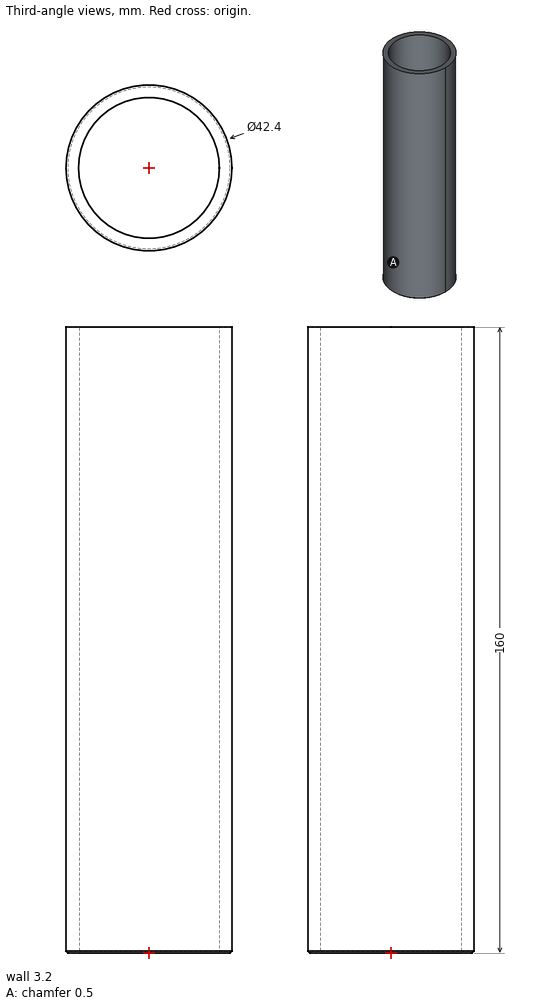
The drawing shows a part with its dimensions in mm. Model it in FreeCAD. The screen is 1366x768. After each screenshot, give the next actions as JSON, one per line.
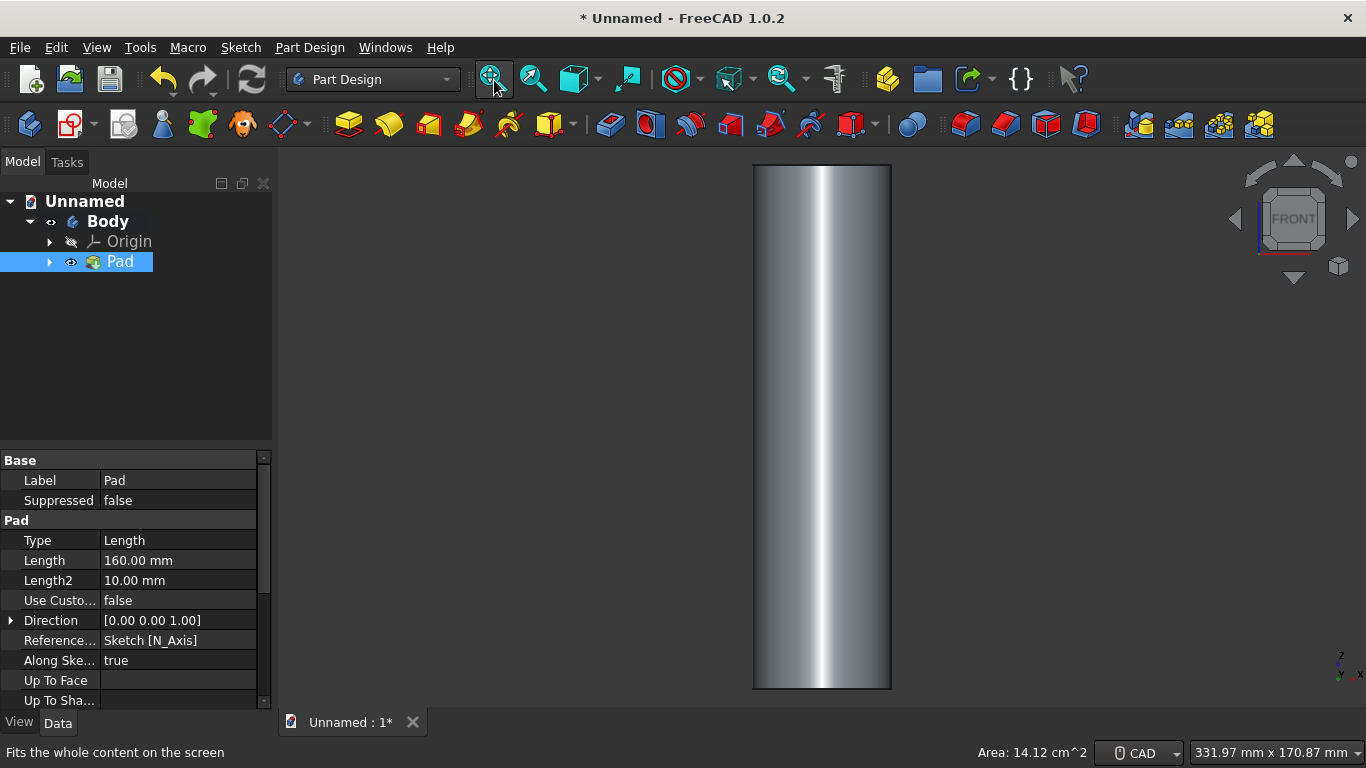
{"action": "key", "text": "3"}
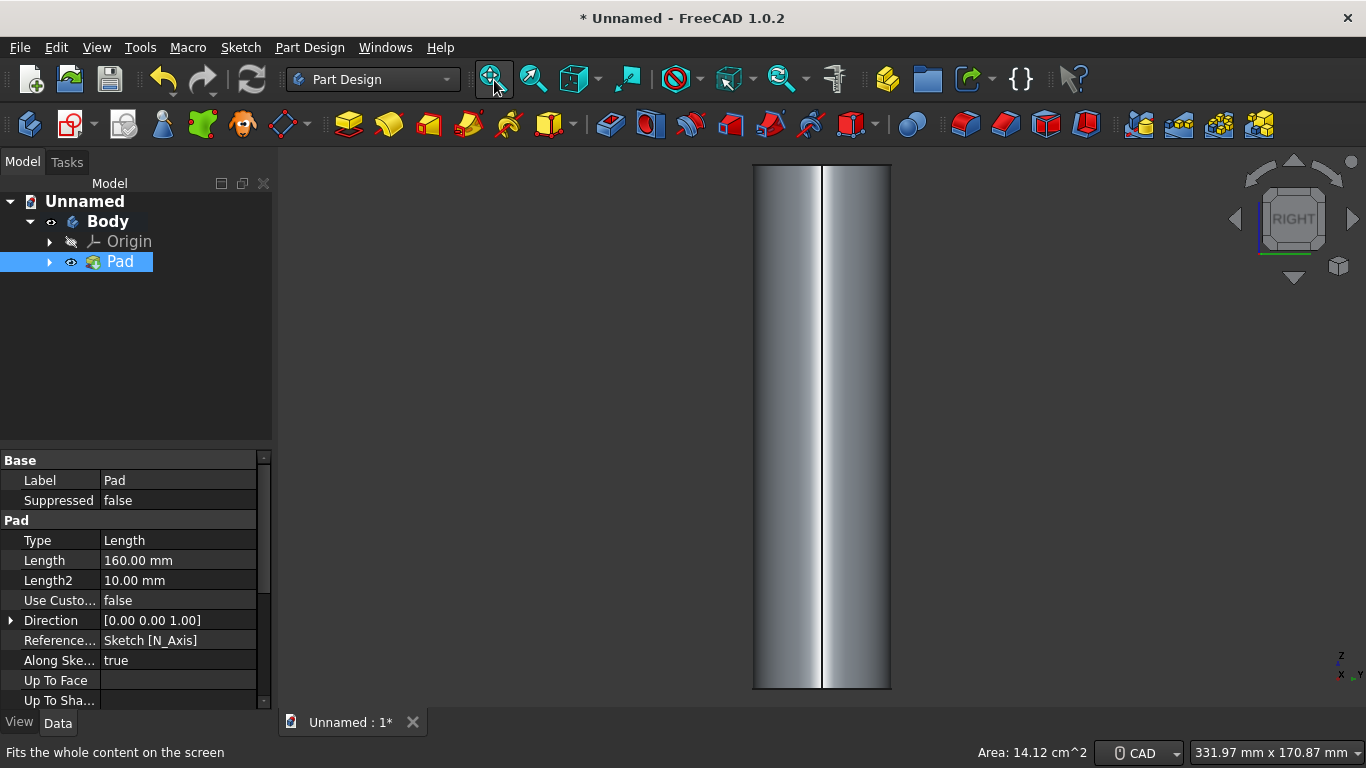
{"action": "key", "text": "5"}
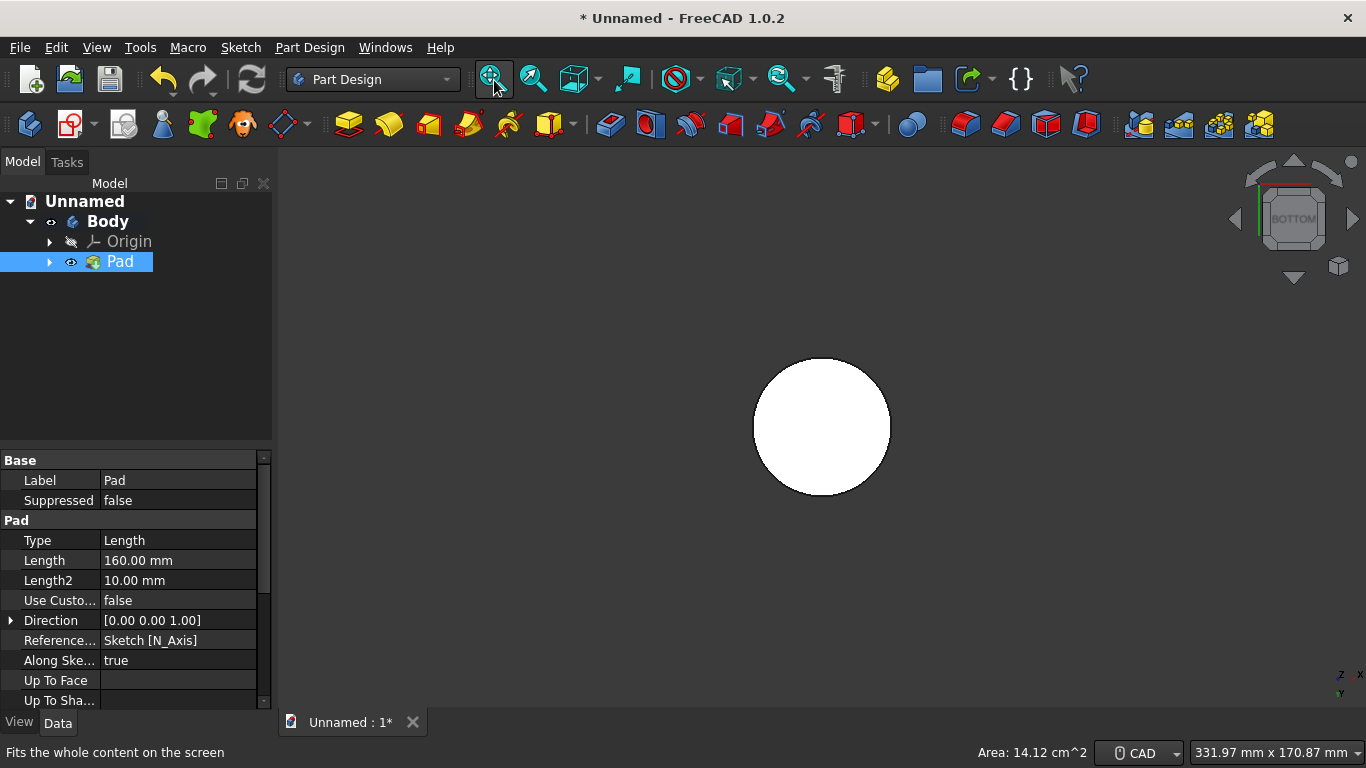
{"action": "left_click", "coordinate": [494, 80]}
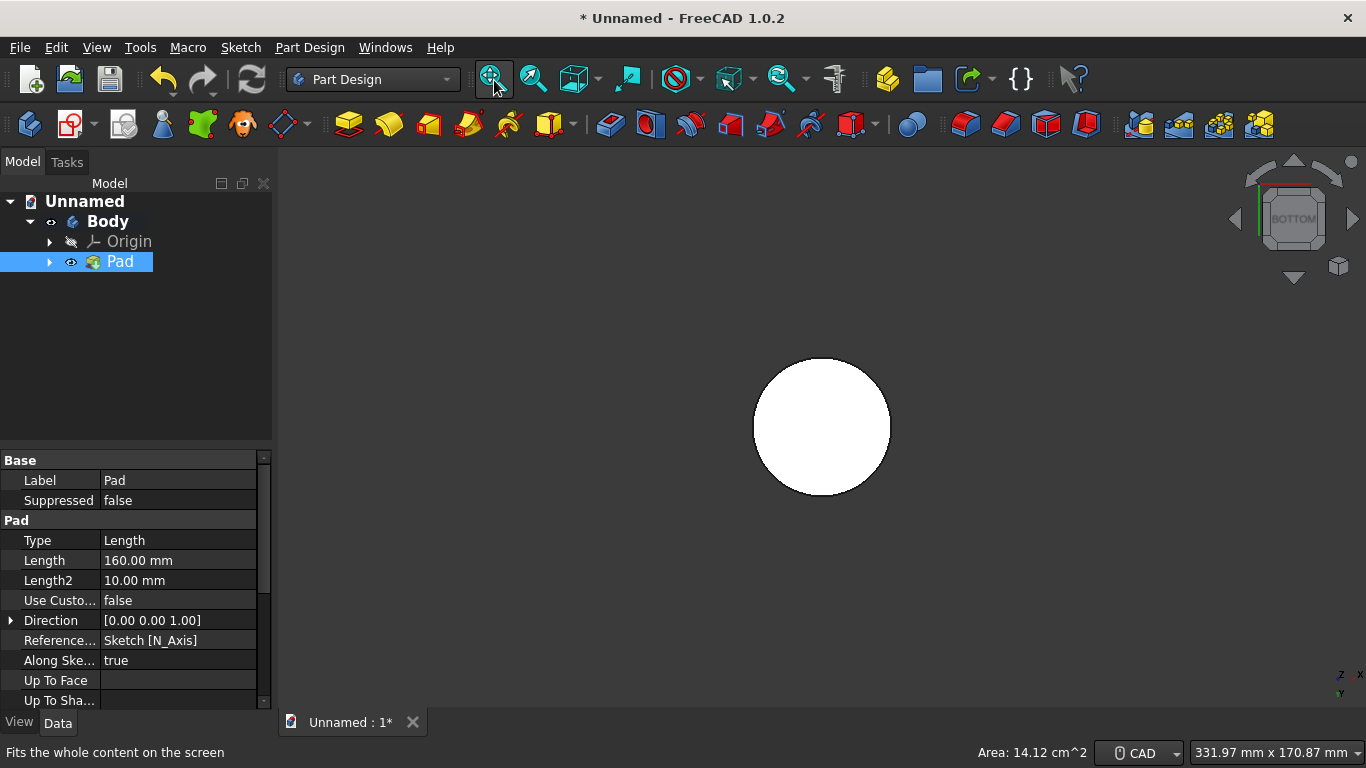
{"action": "left_click", "coordinate": [822, 426], "text": "ctrl"}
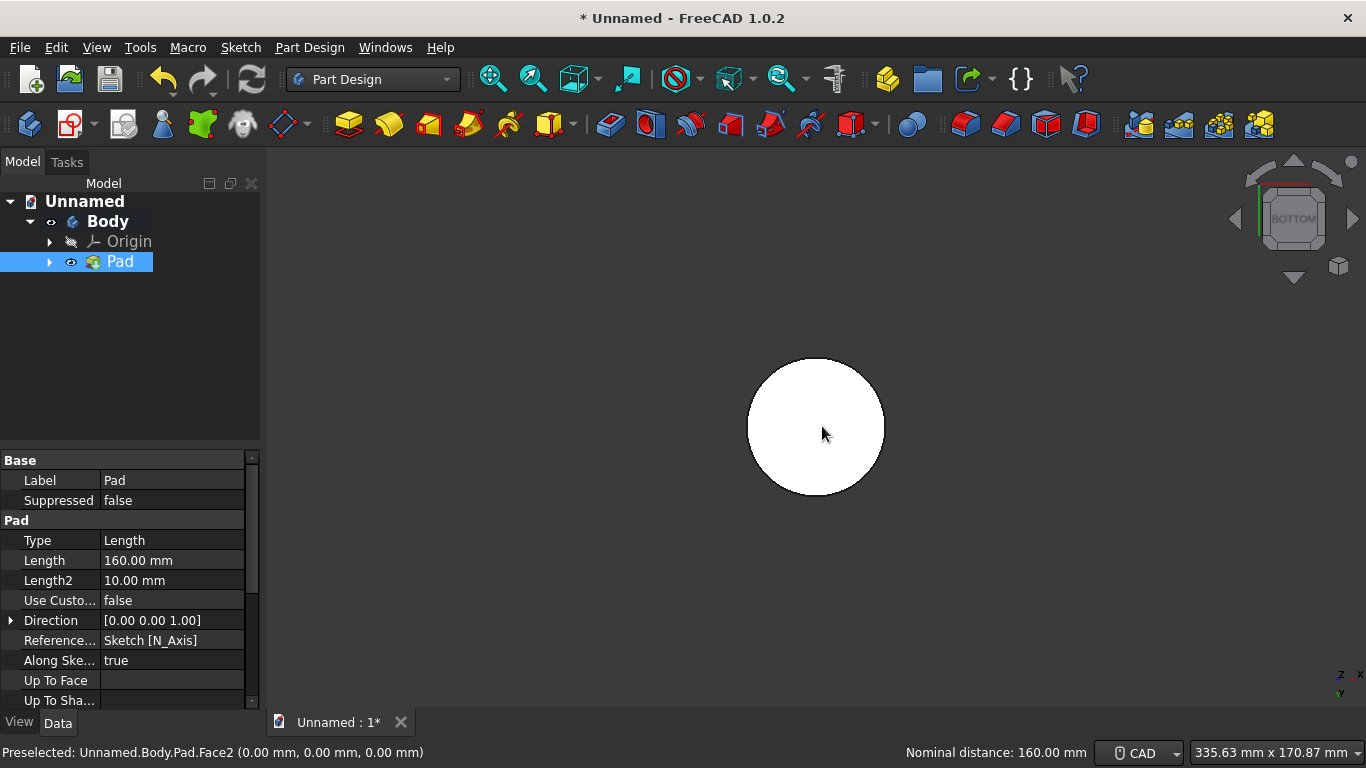
{"action": "left_click", "coordinate": [1086, 124]}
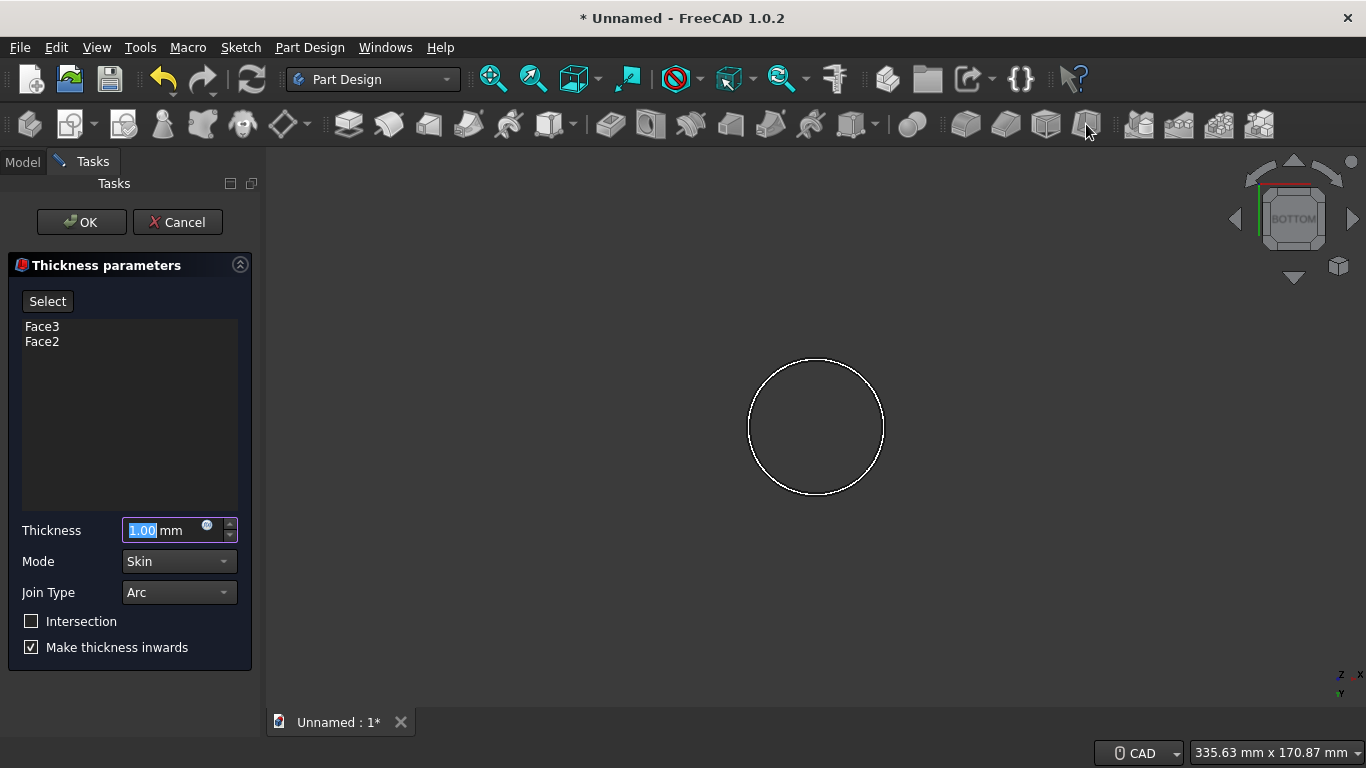
{"action": "type", "text": "3.2"}
{"action": "key", "text": "Tab"}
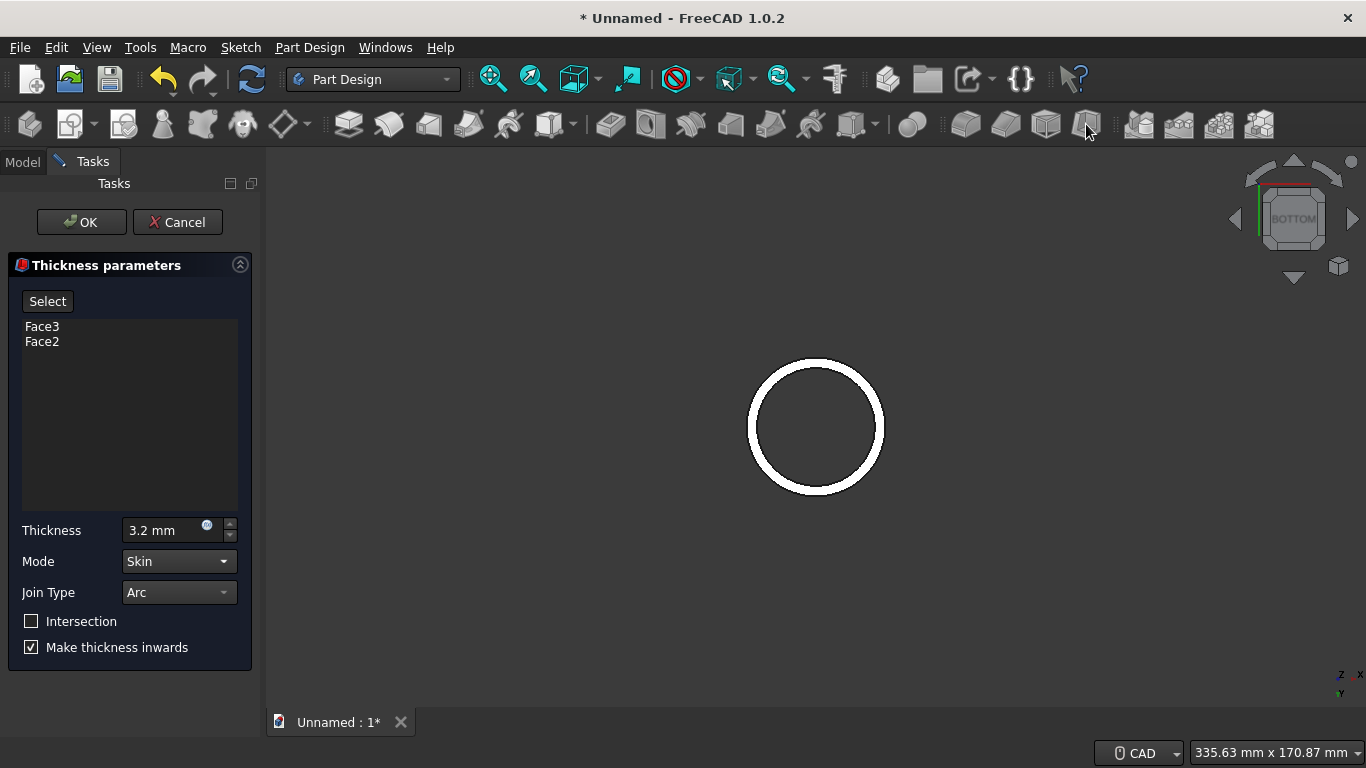
{"action": "left_click", "coordinate": [180, 592]}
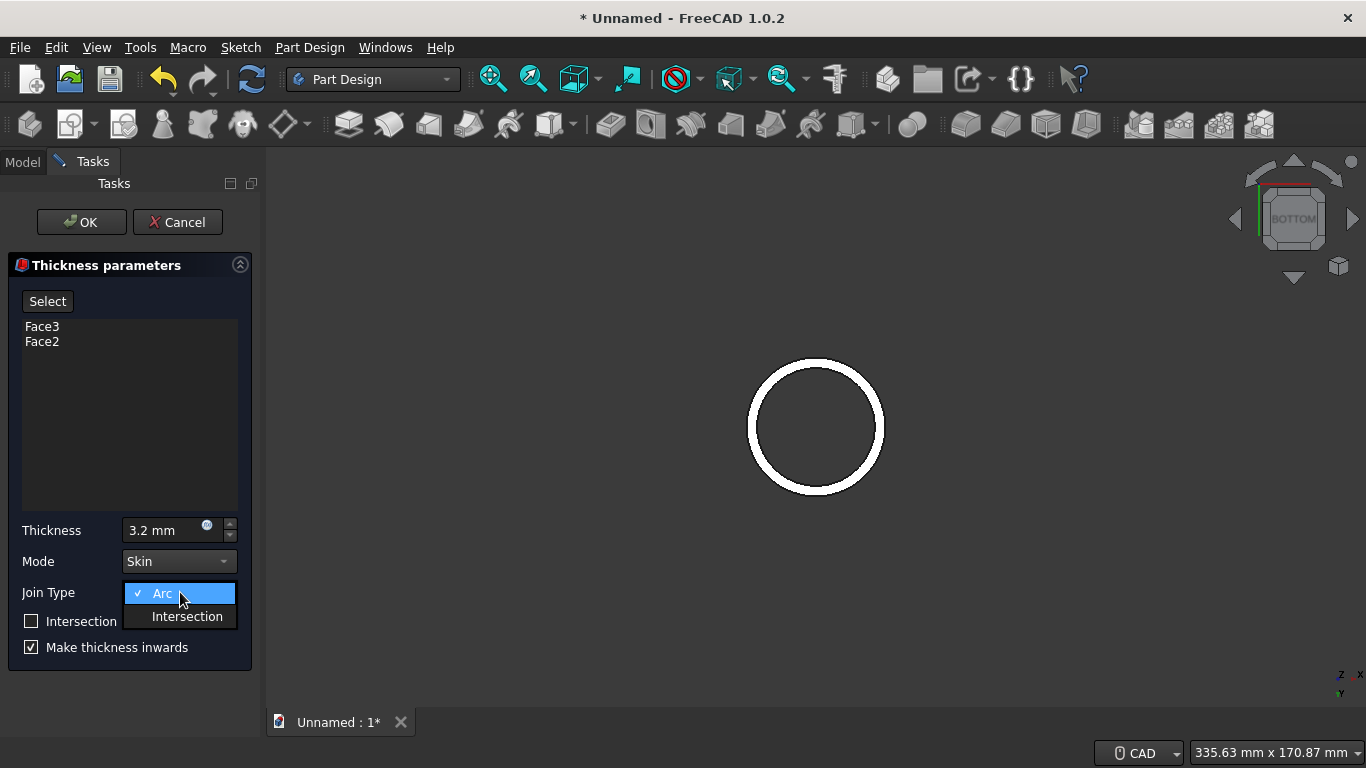
{"action": "left_click", "coordinate": [179, 616]}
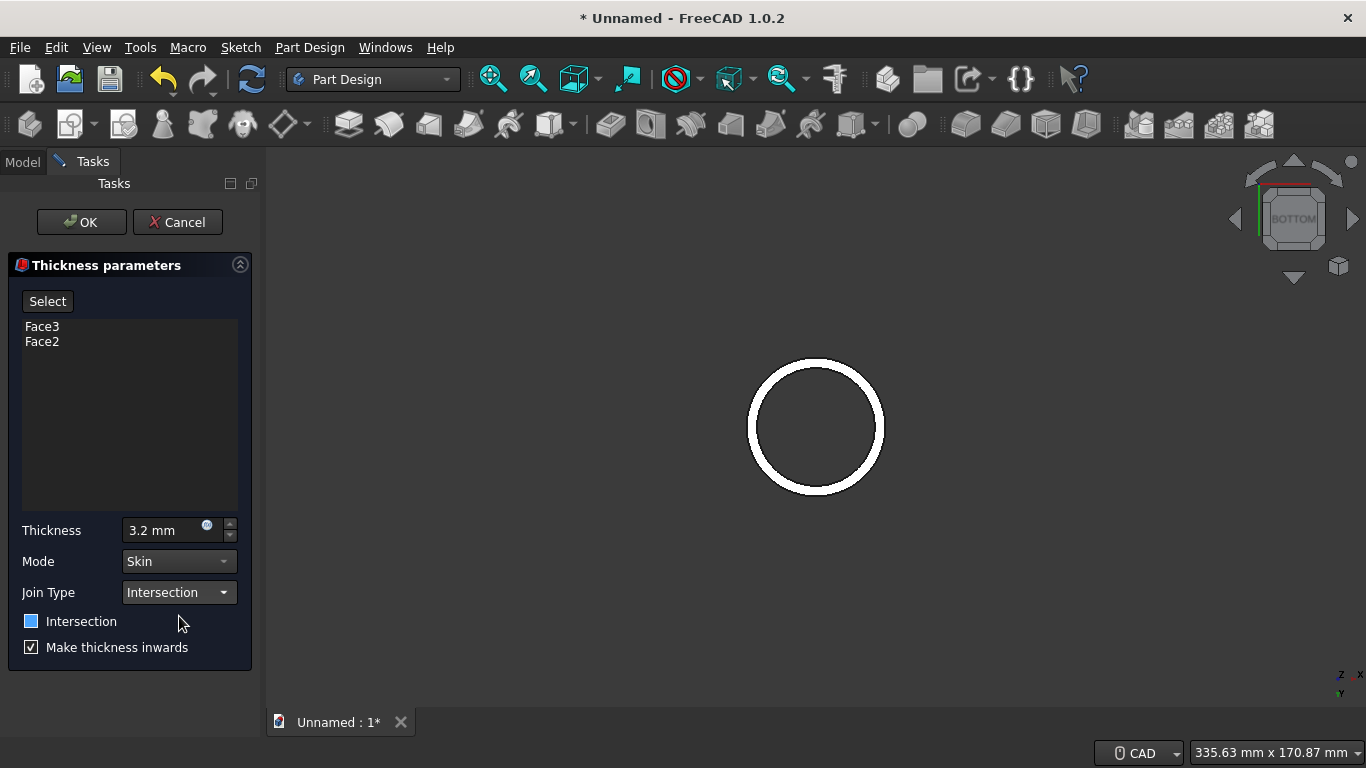
{"action": "left_click", "coordinate": [82, 222]}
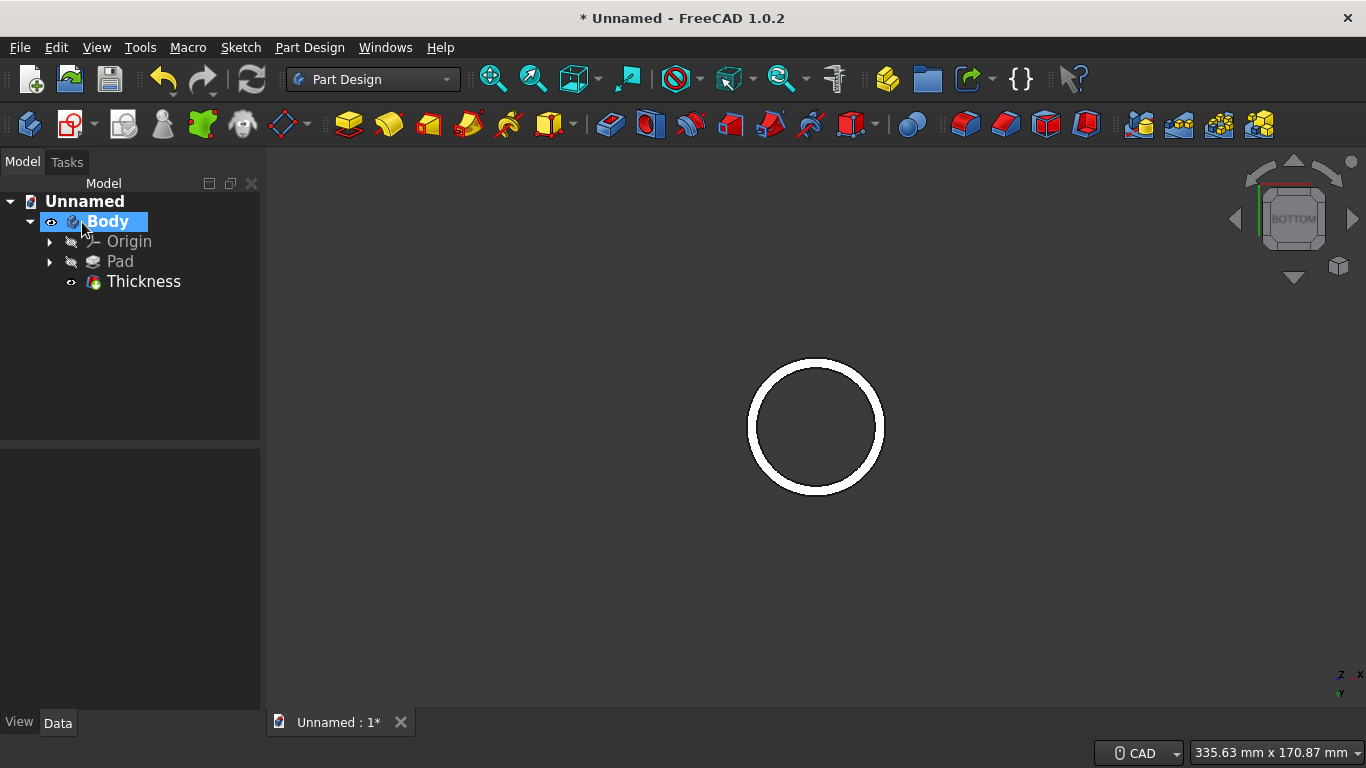
{"action": "left_click", "coordinate": [494, 80]}